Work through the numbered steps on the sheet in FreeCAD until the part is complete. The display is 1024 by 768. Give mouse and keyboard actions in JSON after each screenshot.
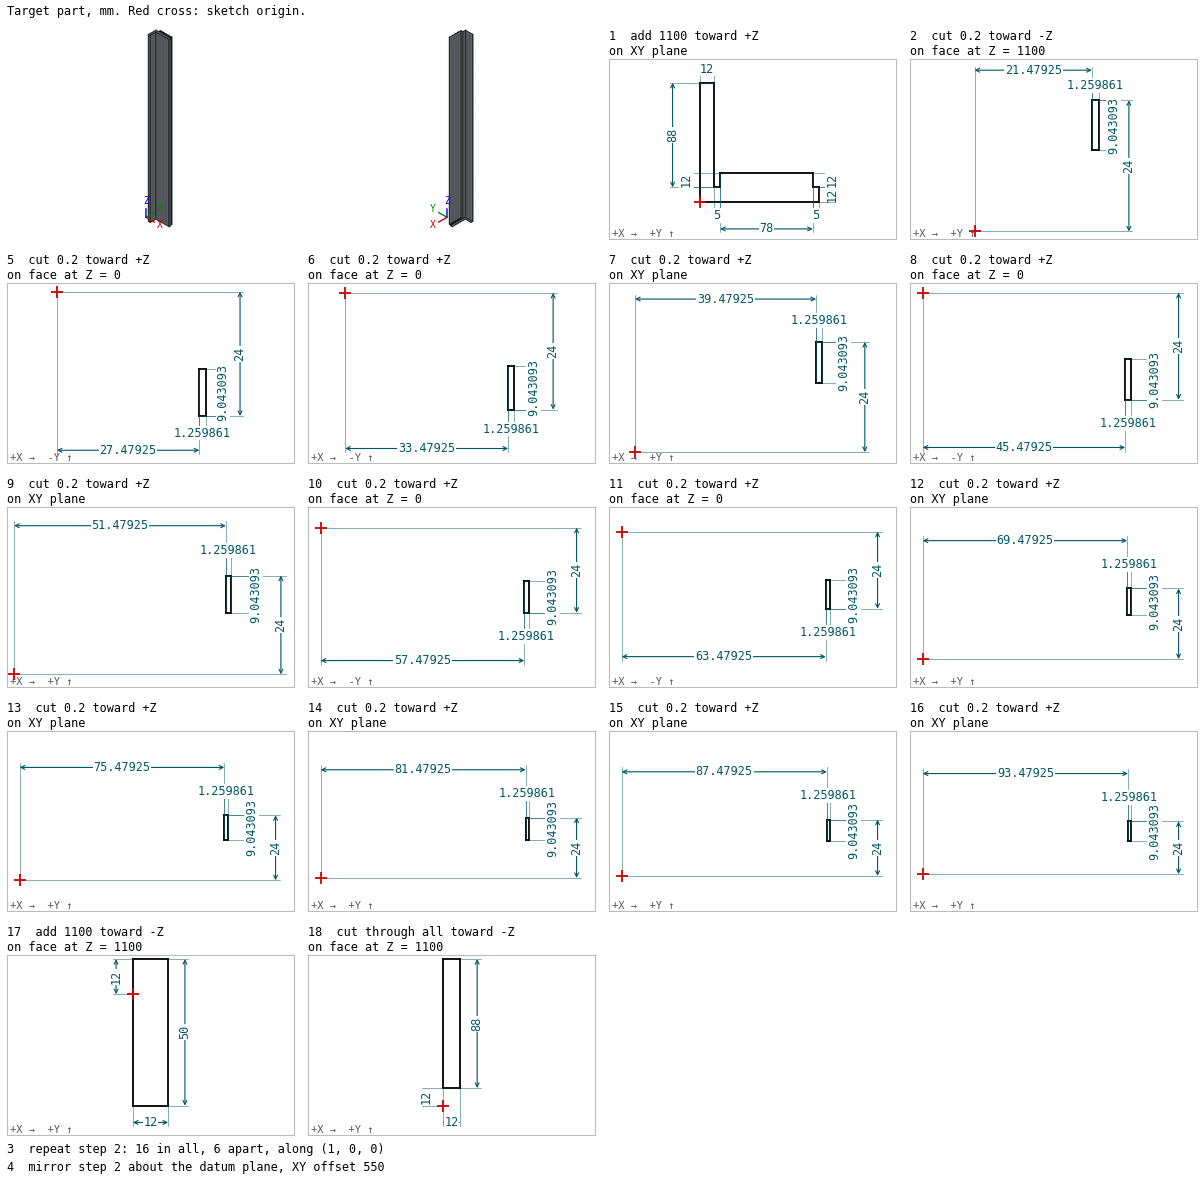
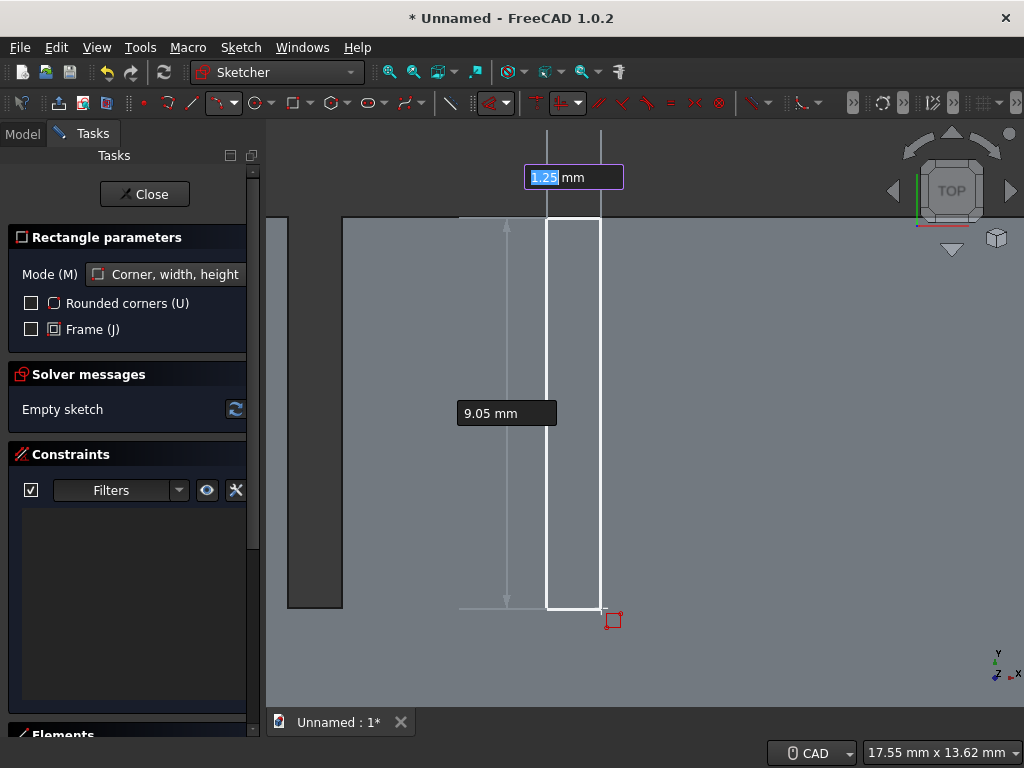
{"action": "type", "text": "1.259861"}
{"action": "key", "text": "Tab"}
{"action": "type", "text": "9.043093"}
{"action": "key", "text": "Return"}
{"action": "key", "text": "Escape"}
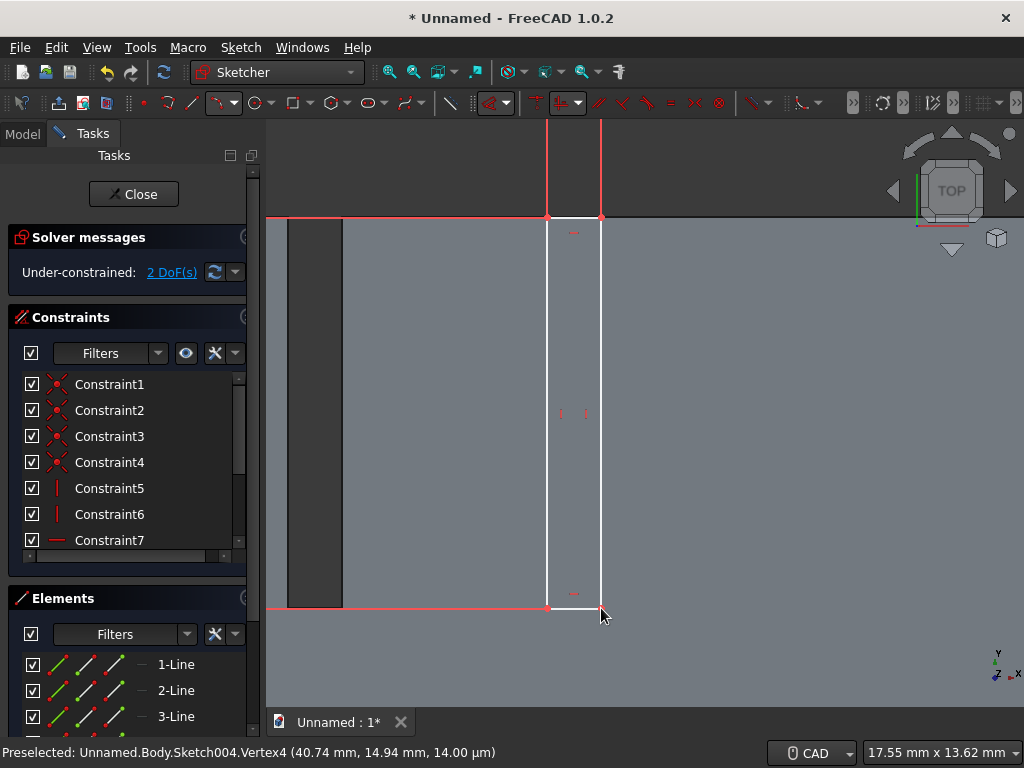
{"action": "left_click", "coordinate": [547, 218]}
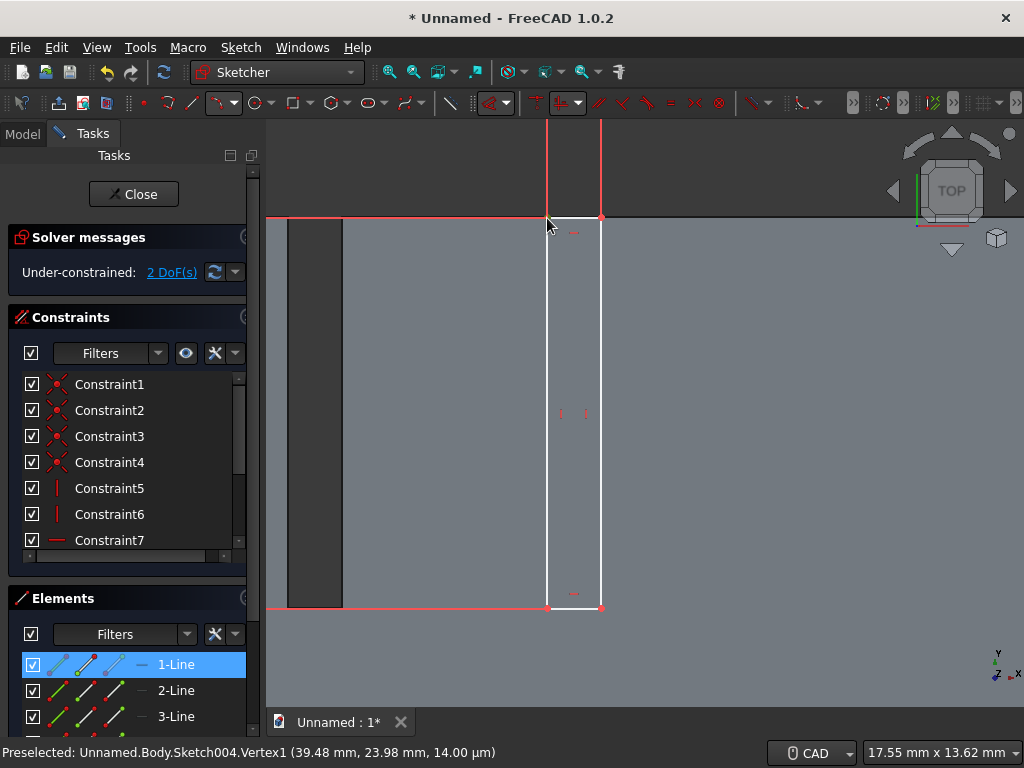
{"action": "left_click", "coordinate": [508, 104]}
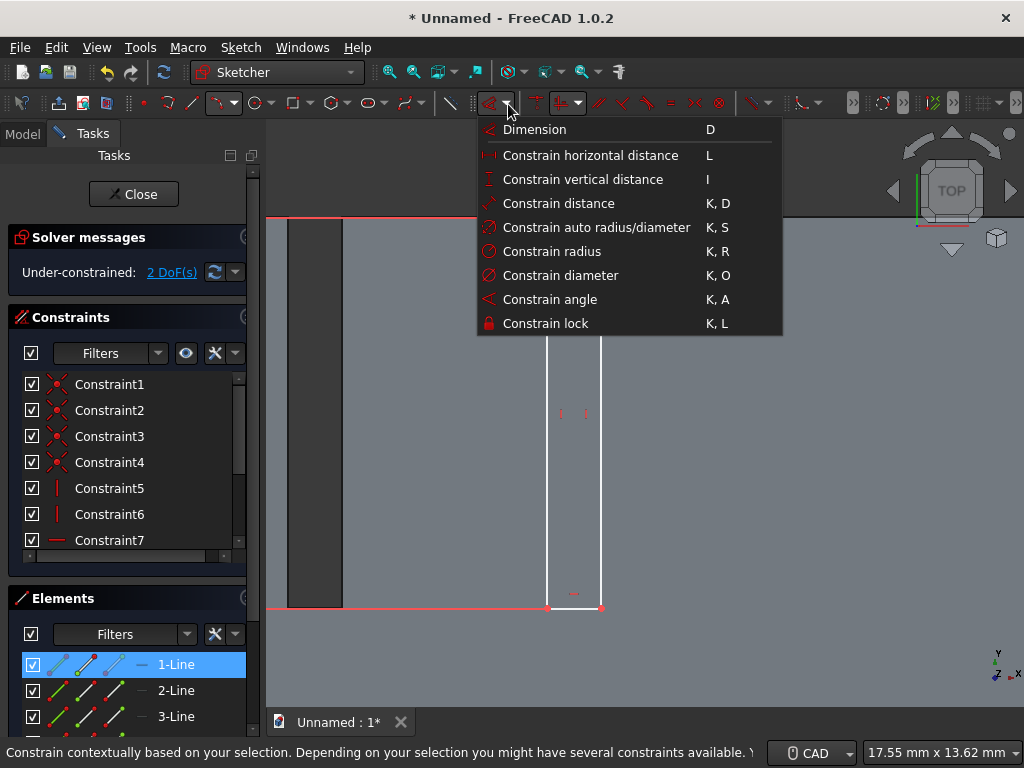
{"action": "left_click", "coordinate": [630, 179]}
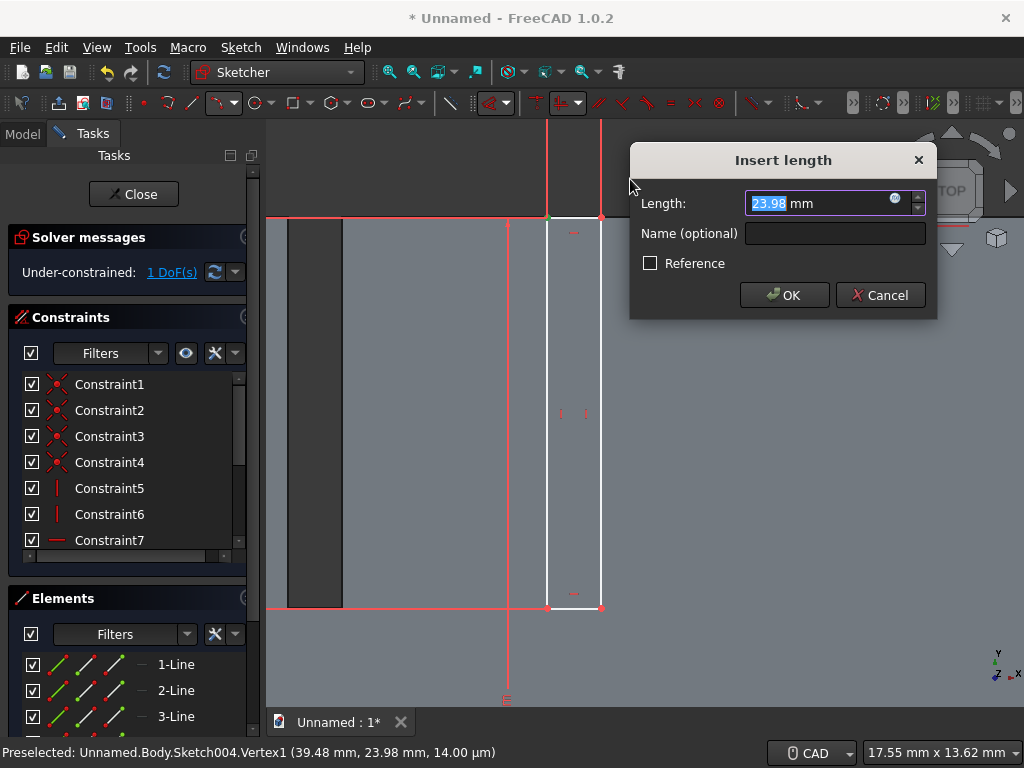
{"action": "type", "text": "24"}
{"action": "key", "text": "Return"}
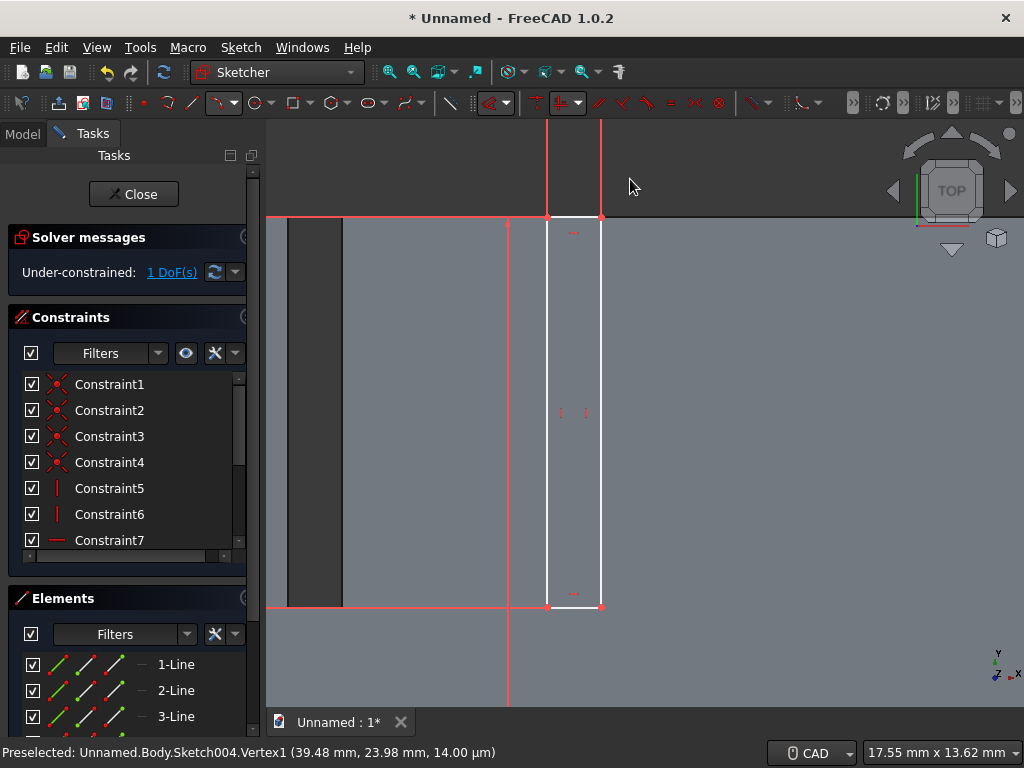
{"action": "left_click", "coordinate": [547, 217]}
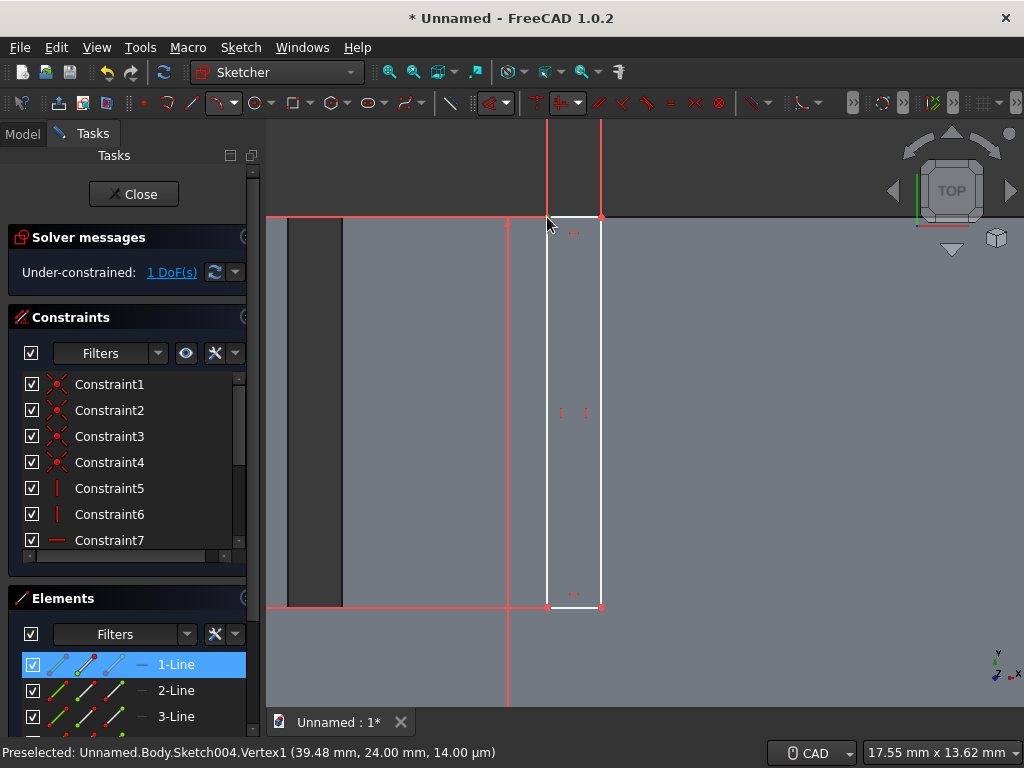
{"action": "key", "text": "l"}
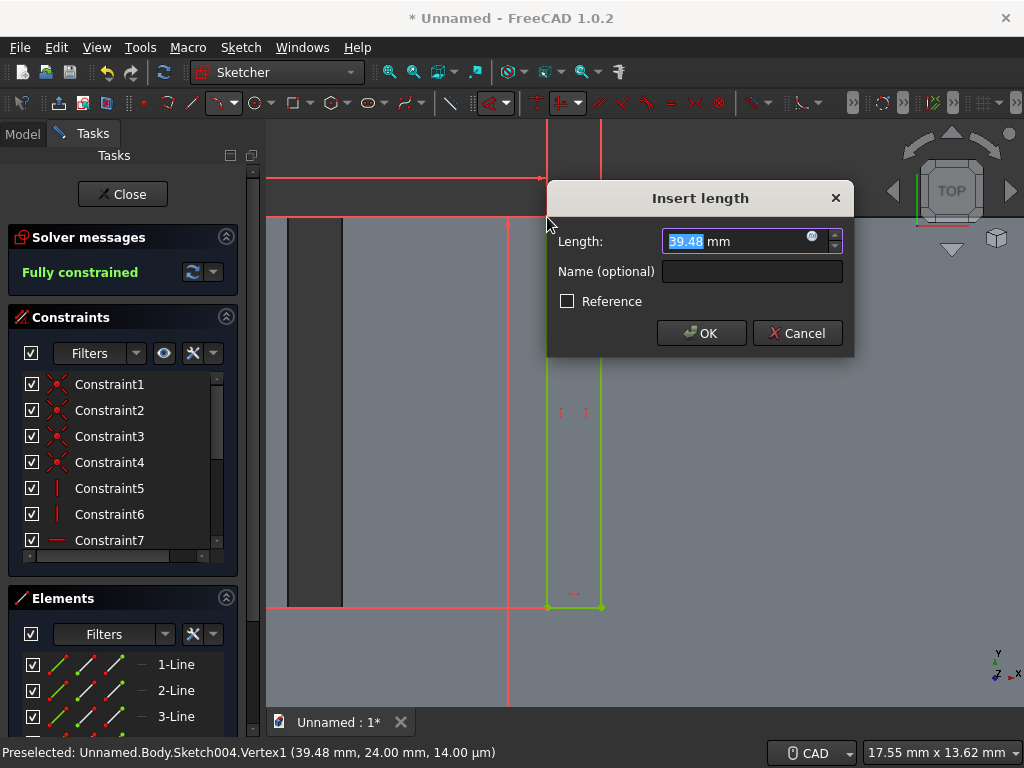
{"action": "type", "text": "39.47925"}
{"action": "key", "text": "Return"}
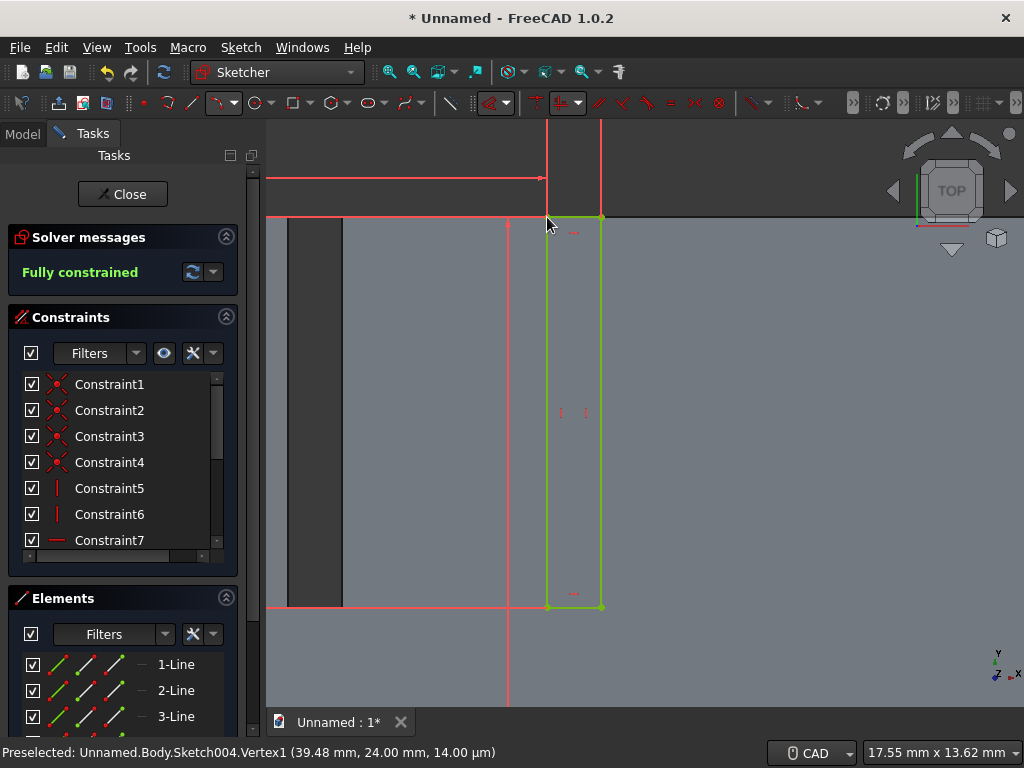
{"action": "left_click", "coordinate": [123, 194]}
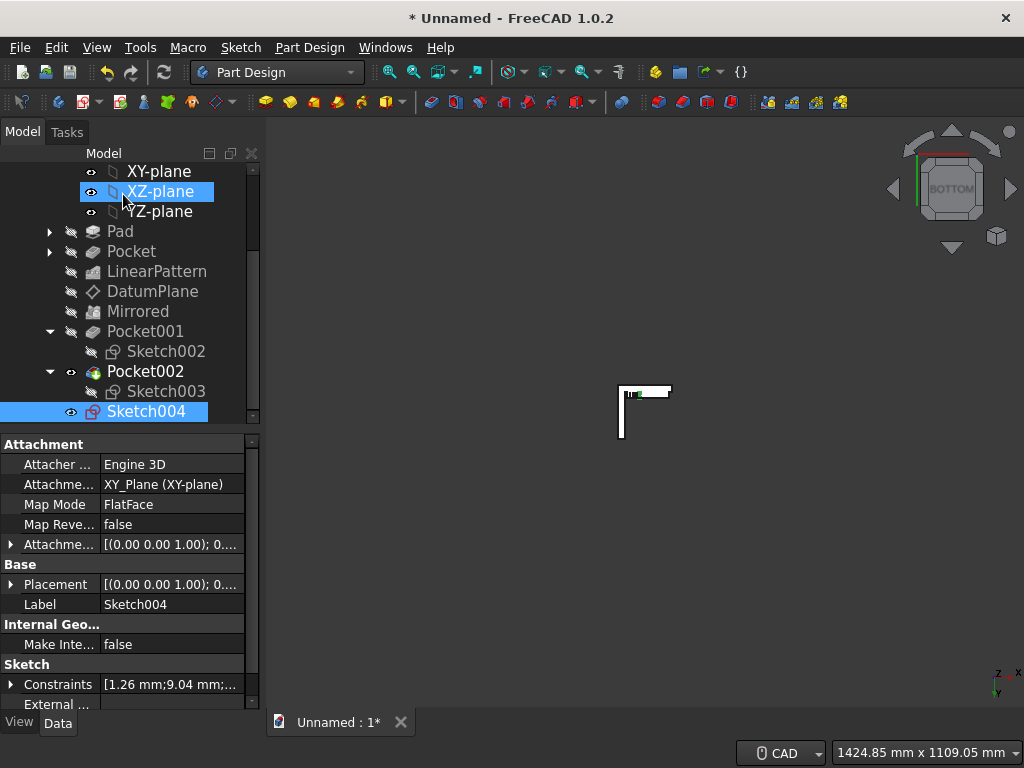
{"action": "left_click", "coordinate": [432, 102]}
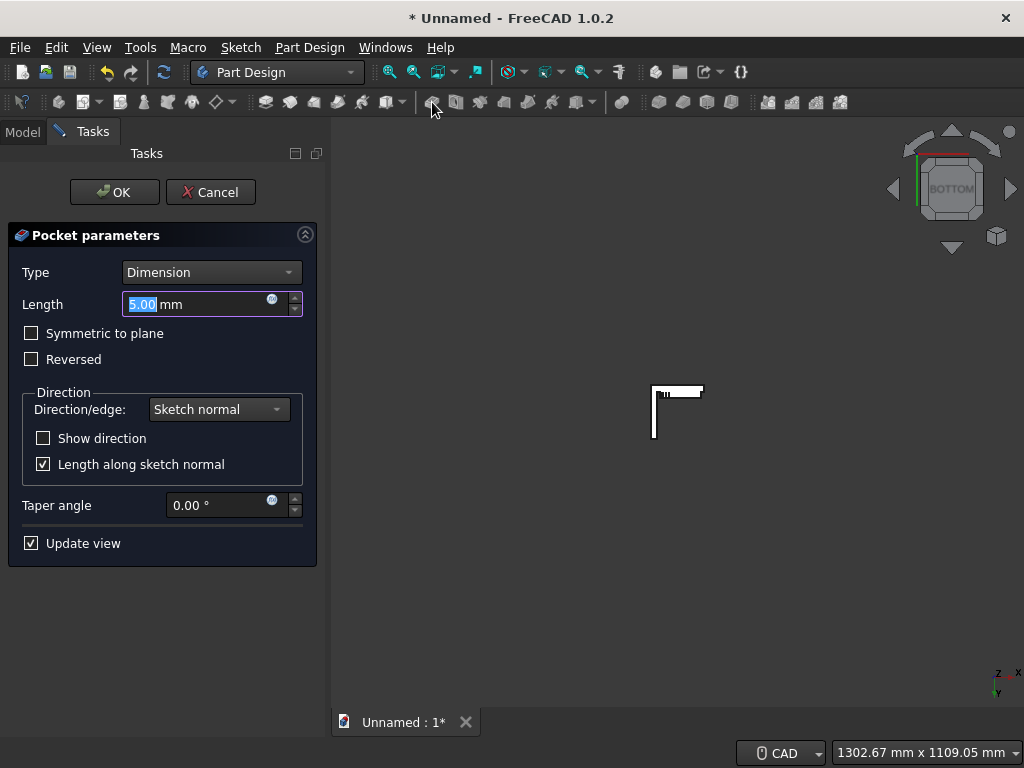
{"action": "type", "text": "0.2"}
{"action": "key", "text": "Tab"}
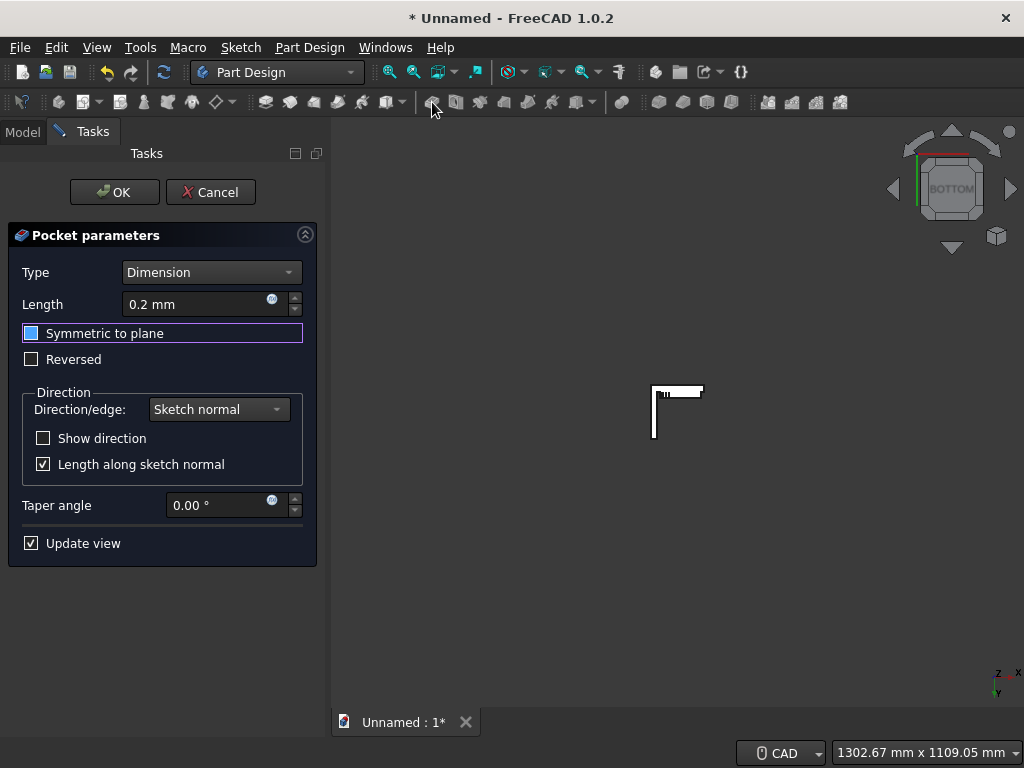
{"action": "left_click", "coordinate": [30, 359]}